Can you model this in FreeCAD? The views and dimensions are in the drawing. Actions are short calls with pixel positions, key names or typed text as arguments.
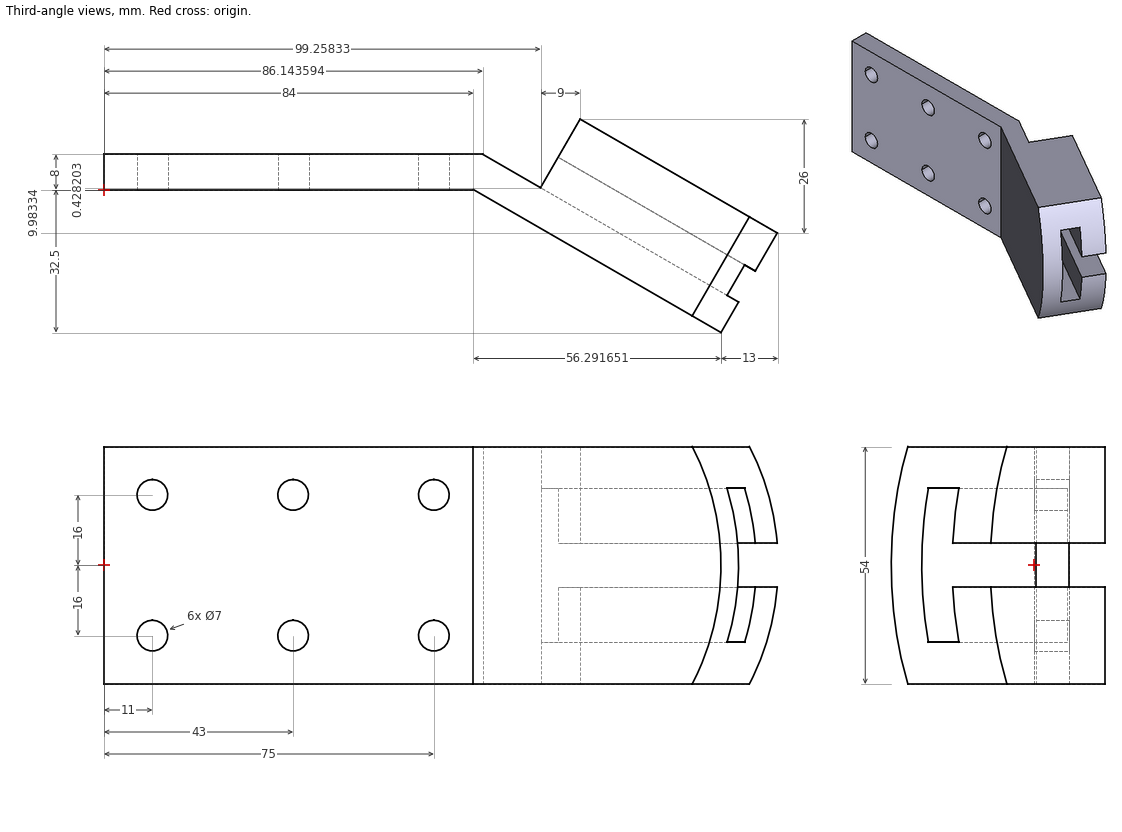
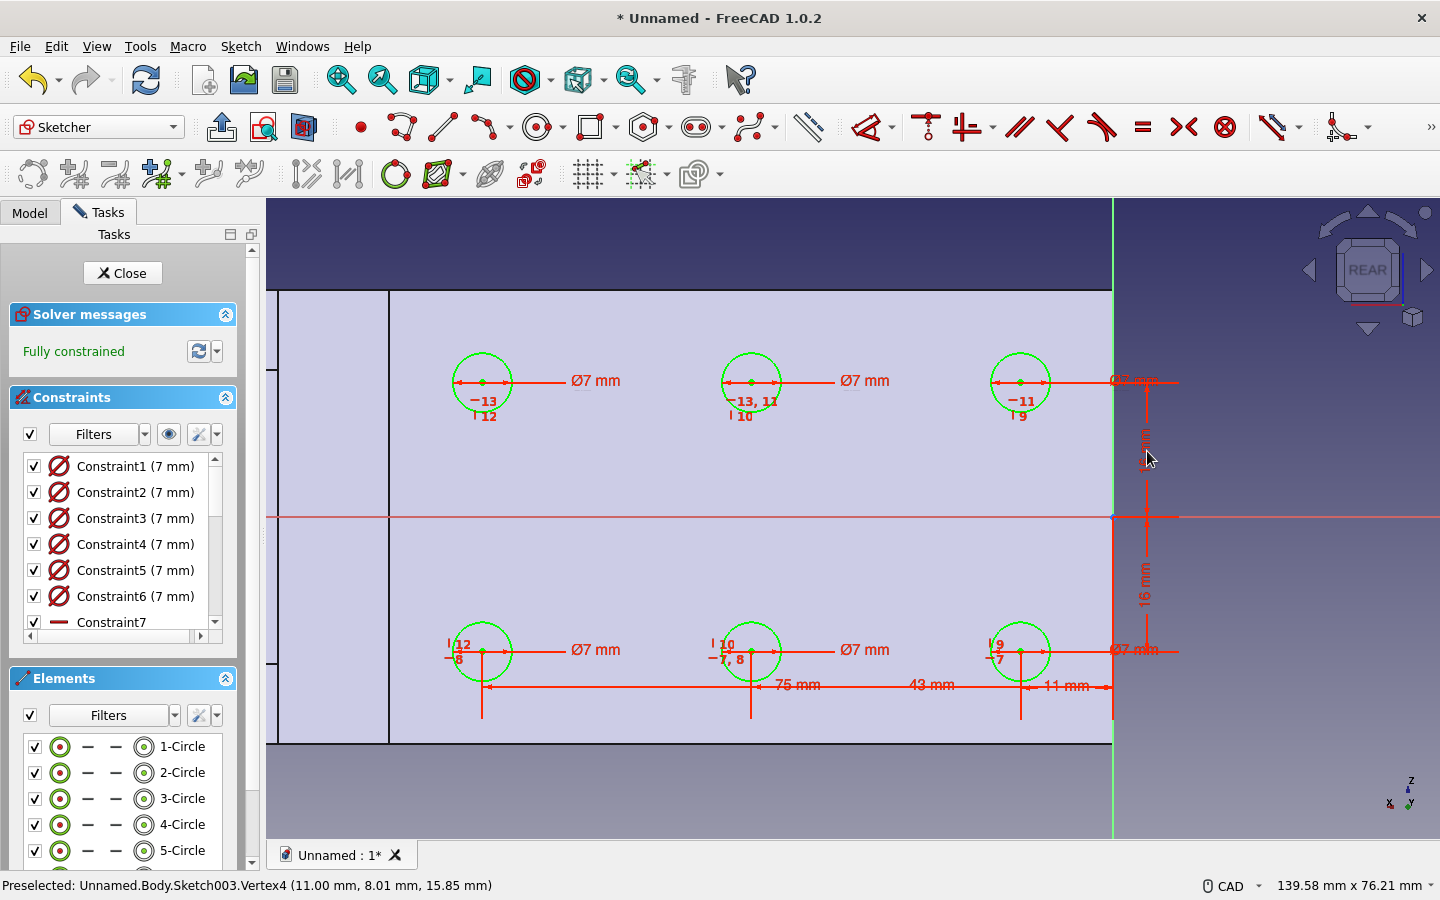
click(123, 273)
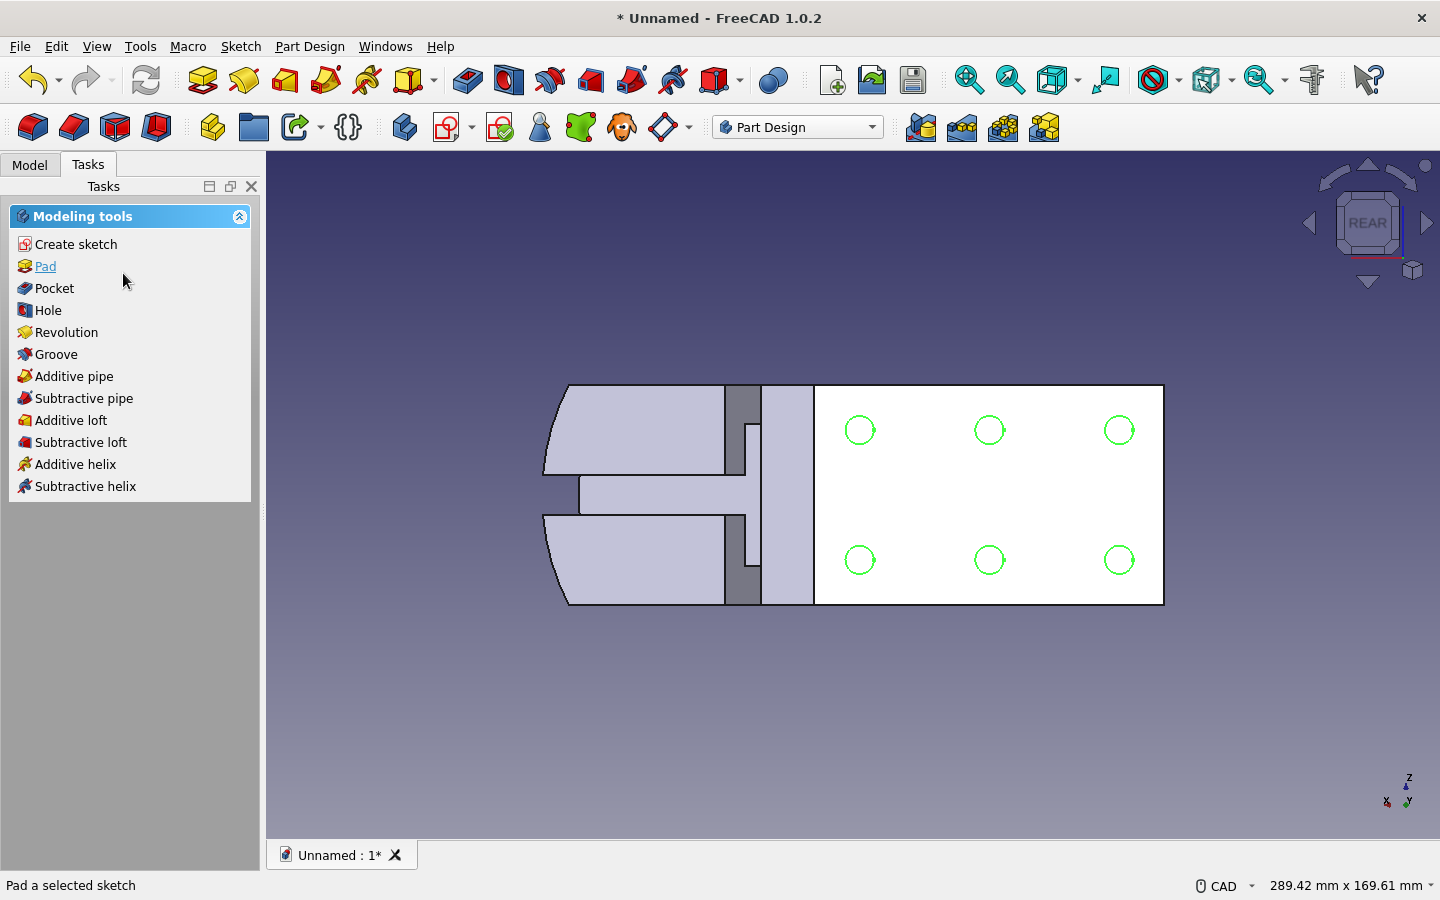
click(468, 80)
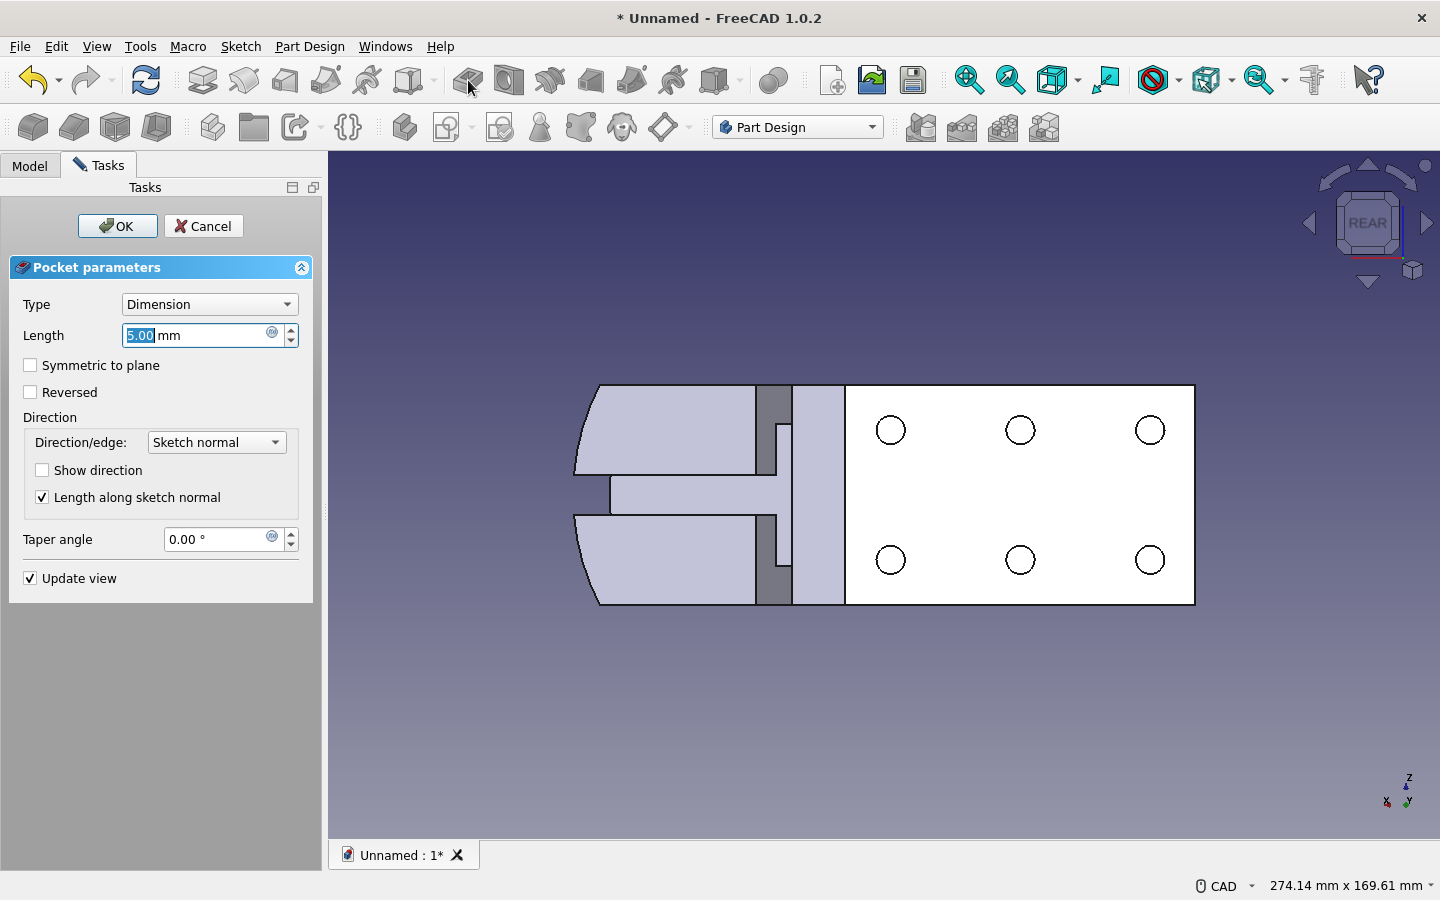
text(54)
key(Tab)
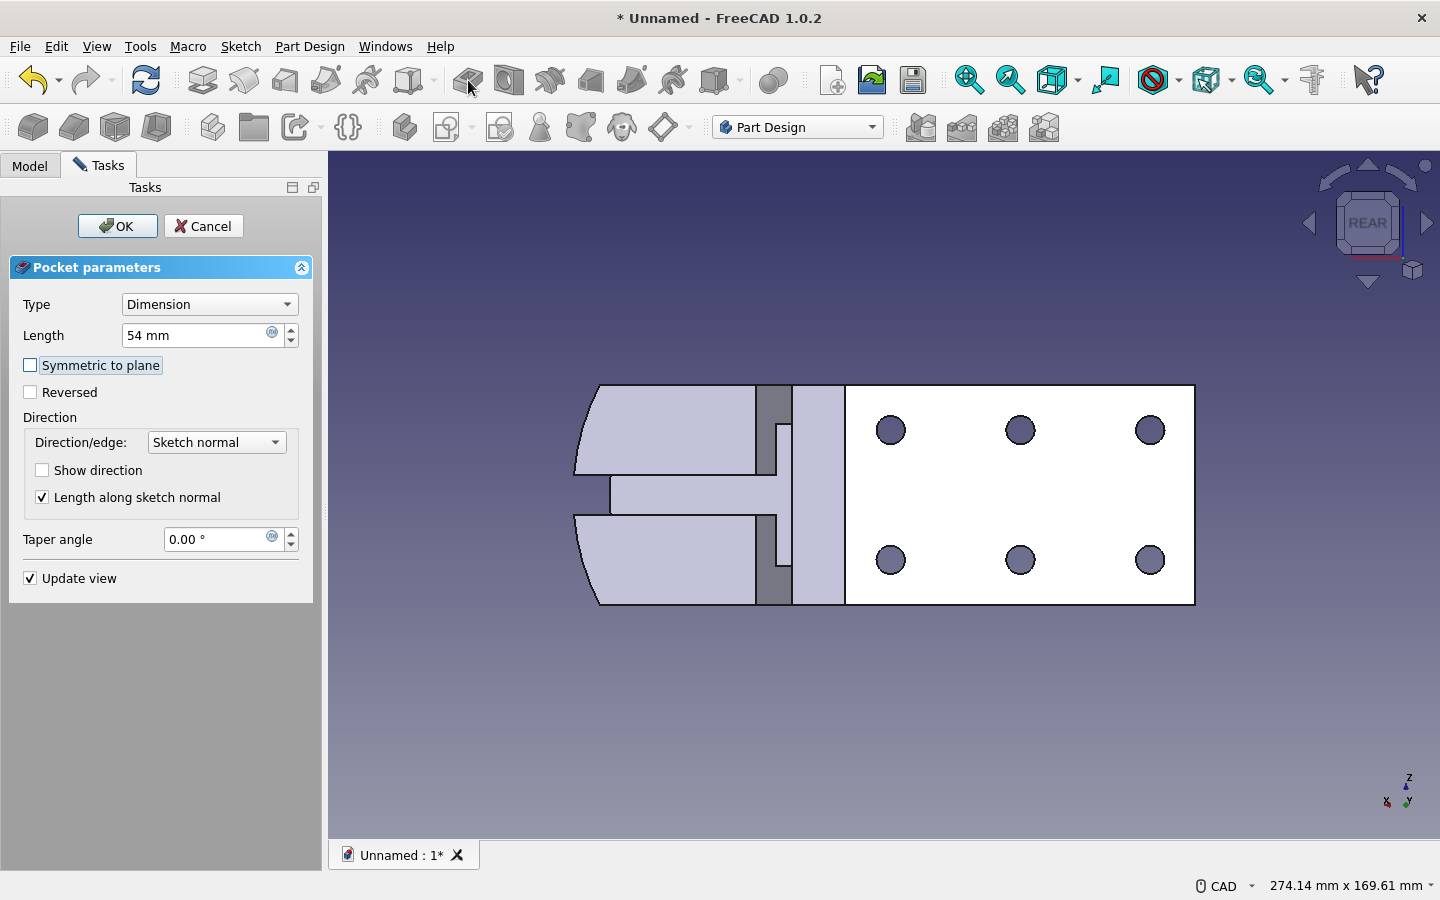
click(118, 226)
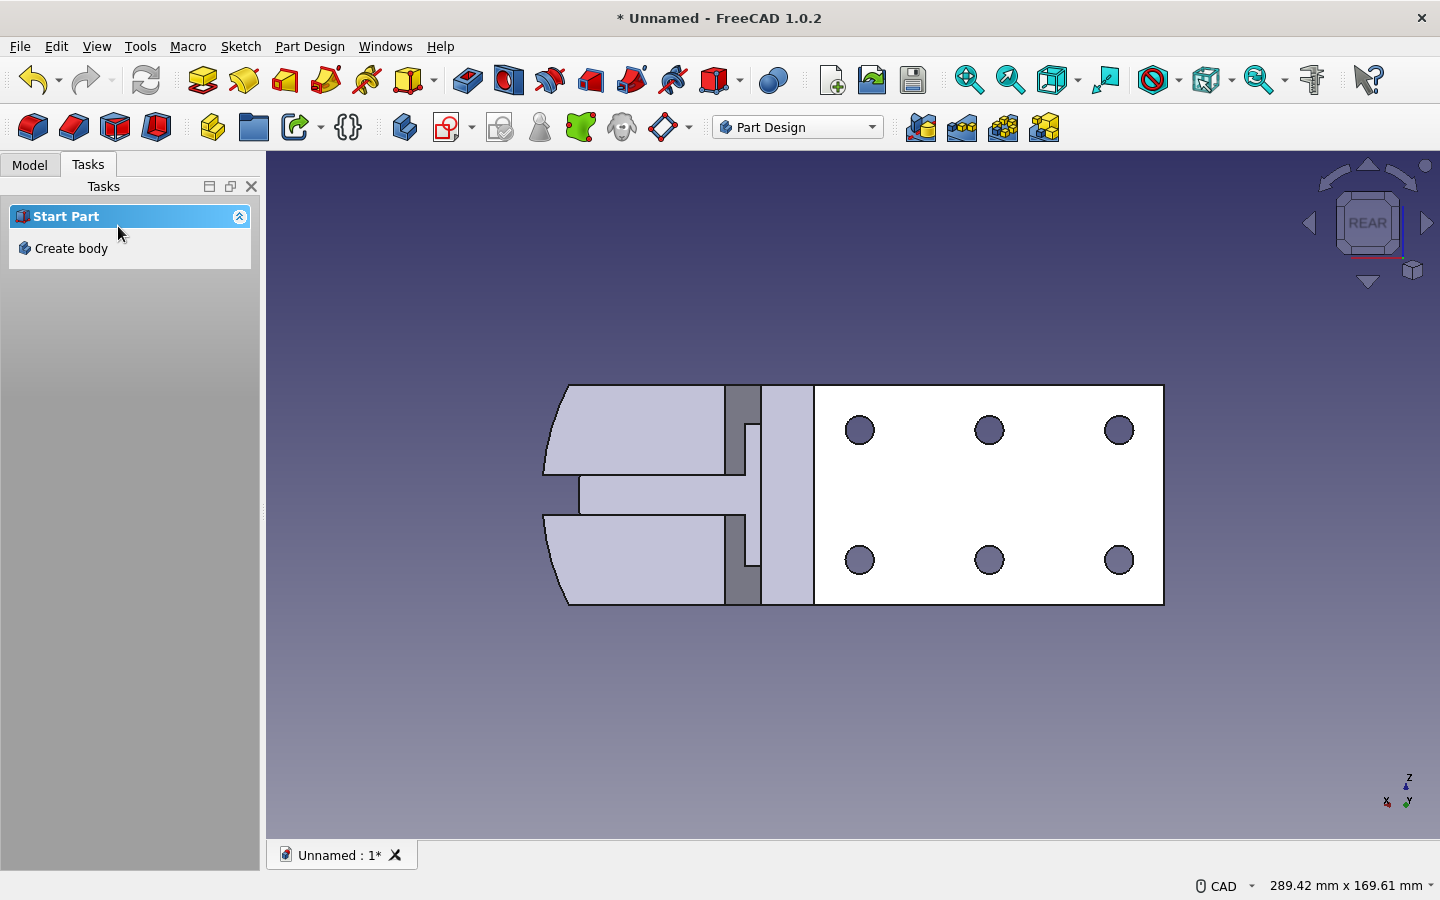
key(0)